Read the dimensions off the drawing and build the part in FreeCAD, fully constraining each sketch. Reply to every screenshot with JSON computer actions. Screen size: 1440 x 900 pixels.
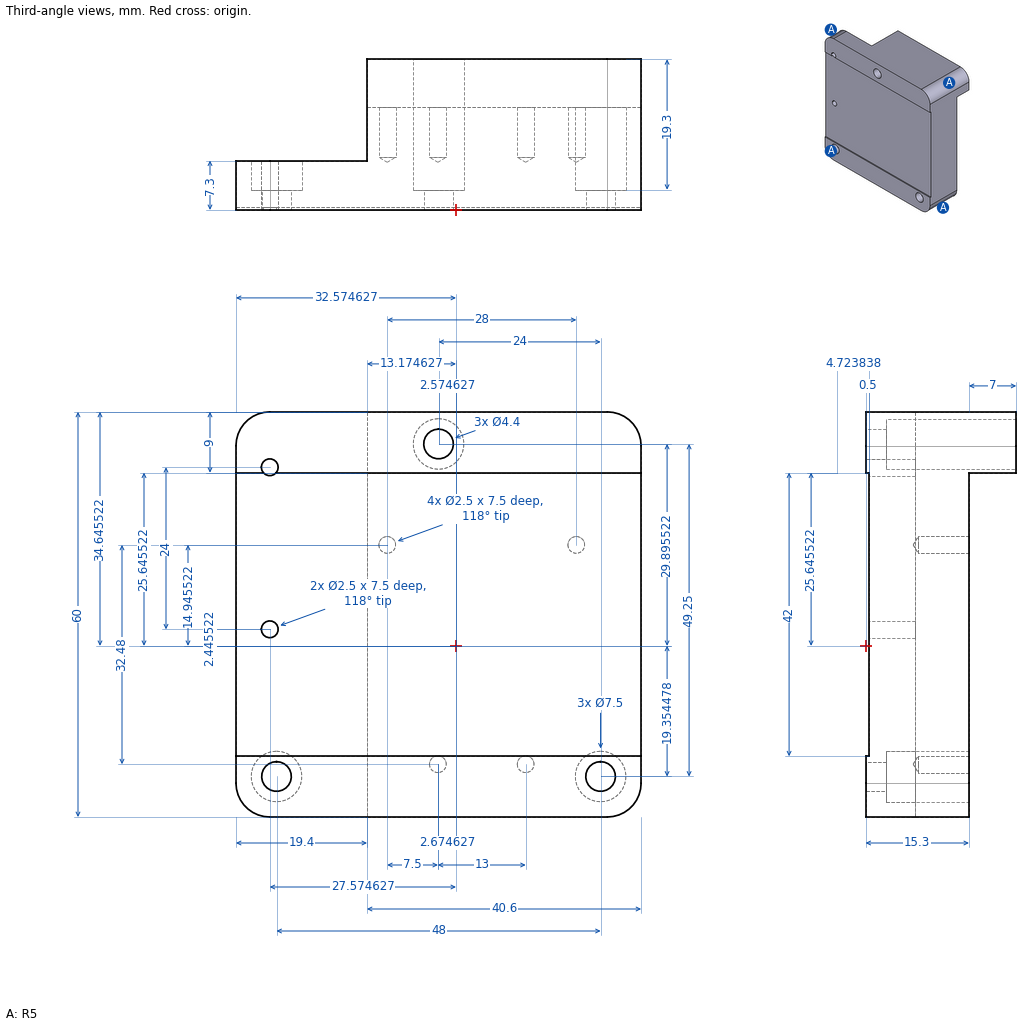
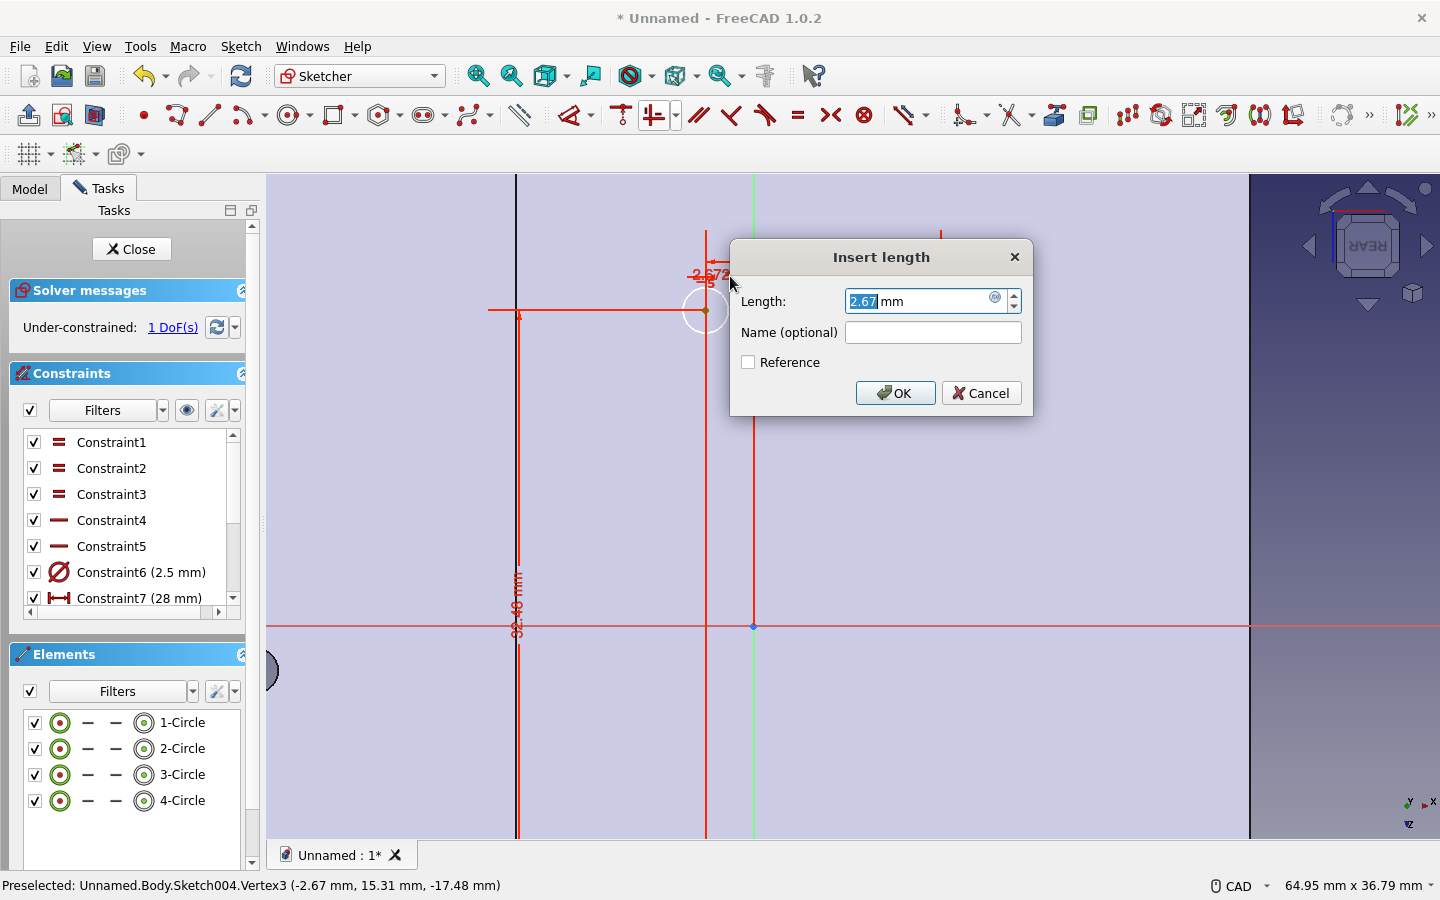
{"action": "type", "text": "2.674627"}
{"action": "key", "text": "Return"}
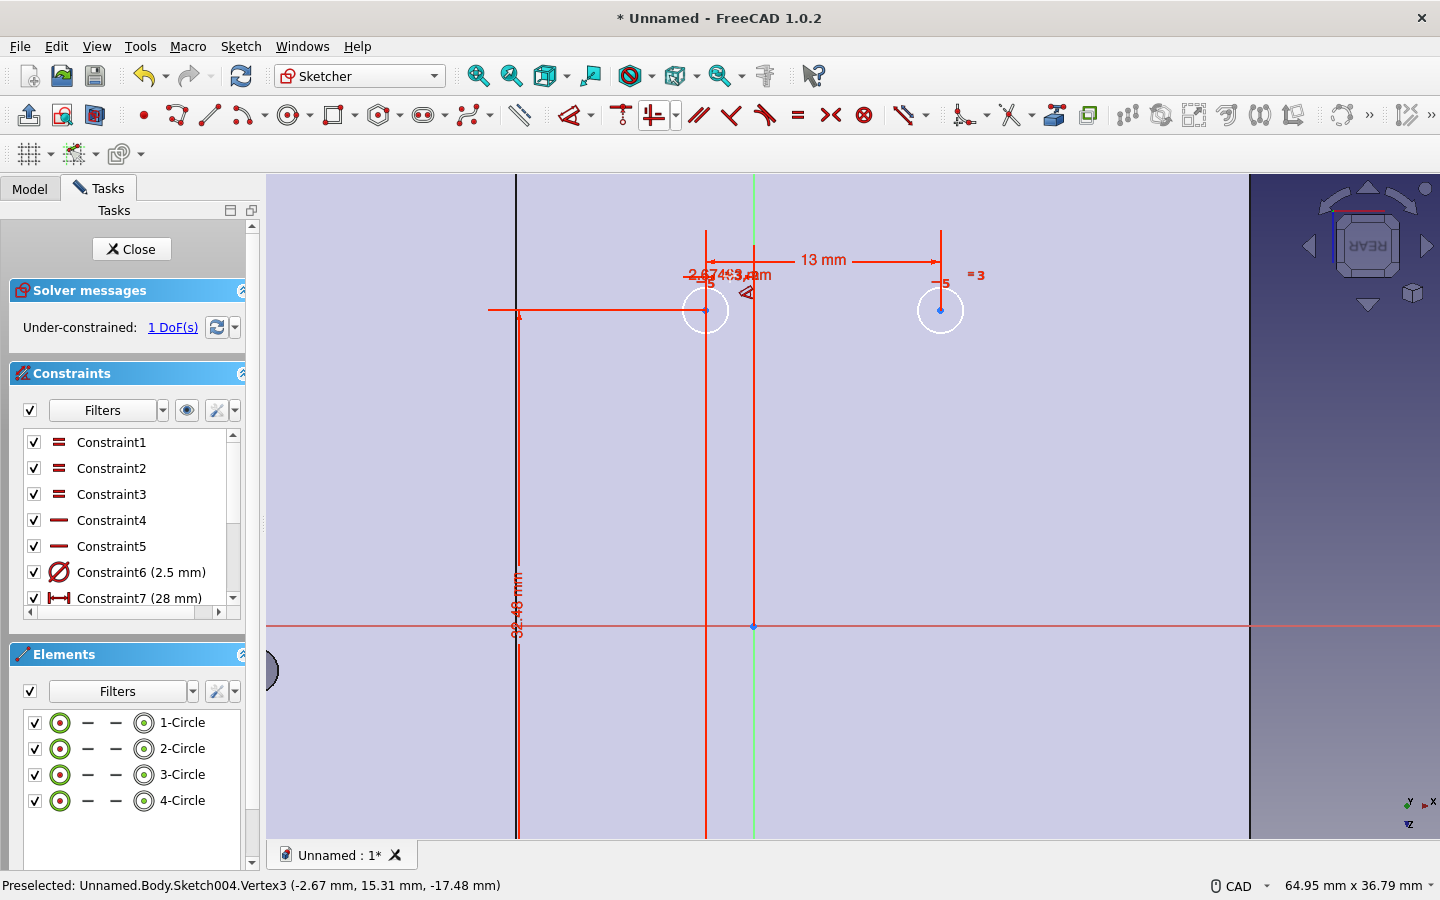
{"action": "scroll", "coordinate": [706, 310], "scroll_direction": "down", "scroll_amount": 2}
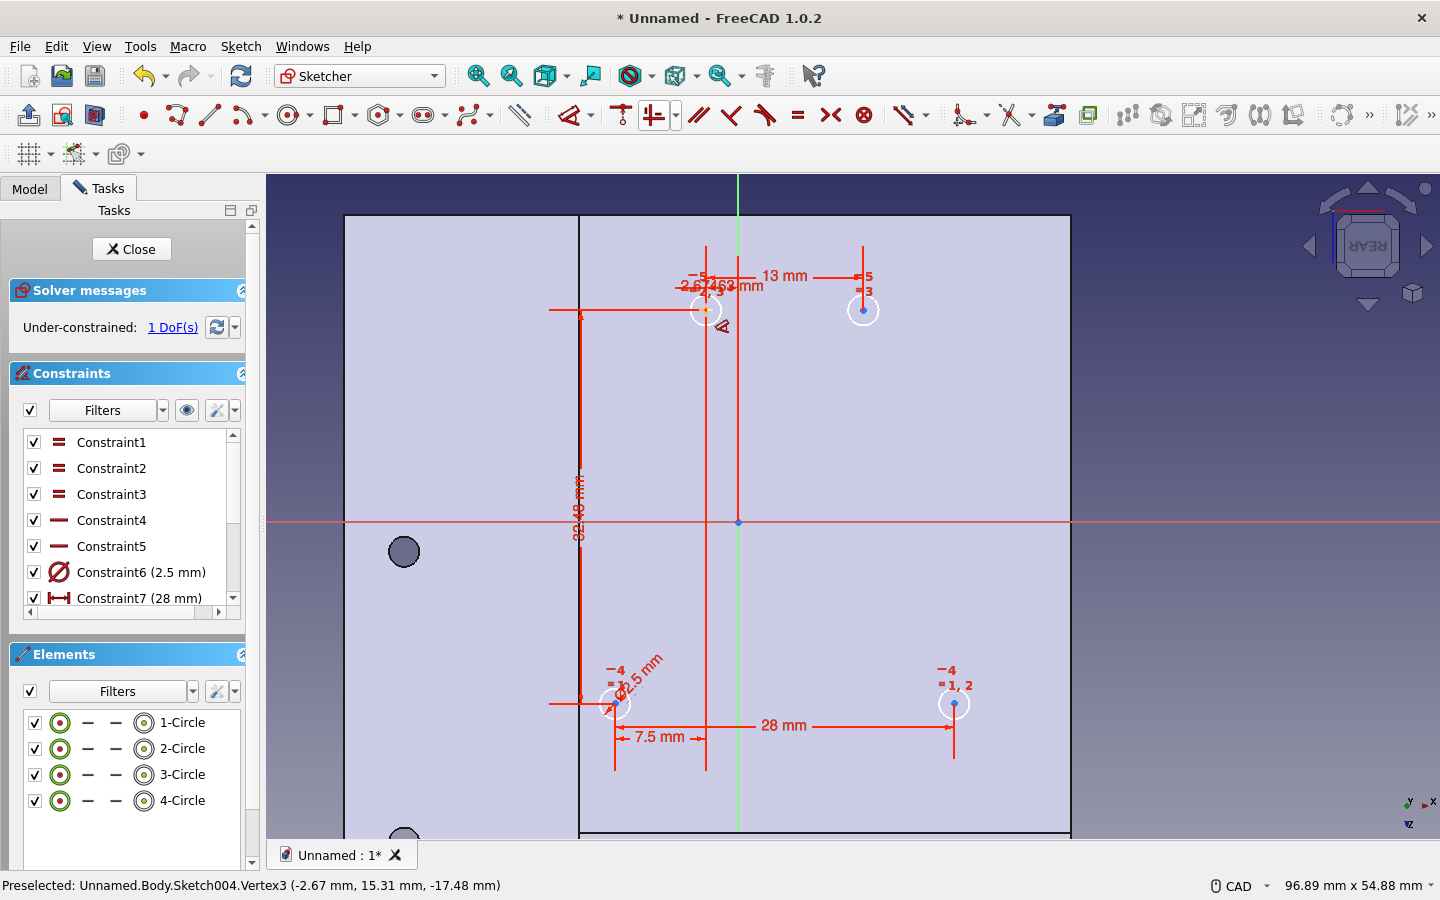
{"action": "left_click", "coordinate": [615, 704]}
{"action": "left_click", "coordinate": [581, 613]}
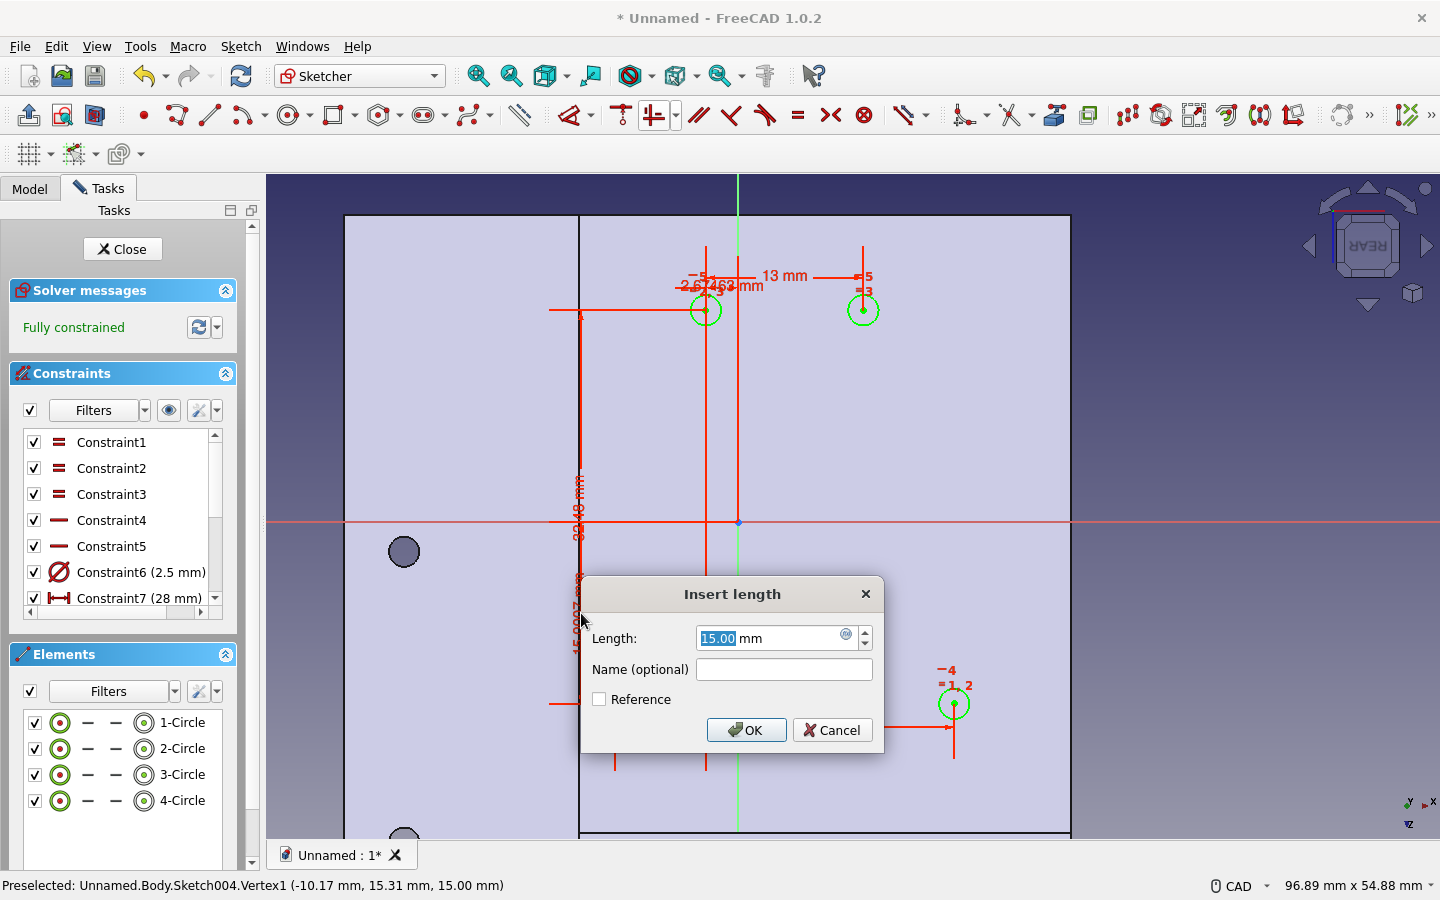
{"action": "type", "text": "14.945522"}
{"action": "key", "text": "Return"}
{"action": "key", "text": "Escape"}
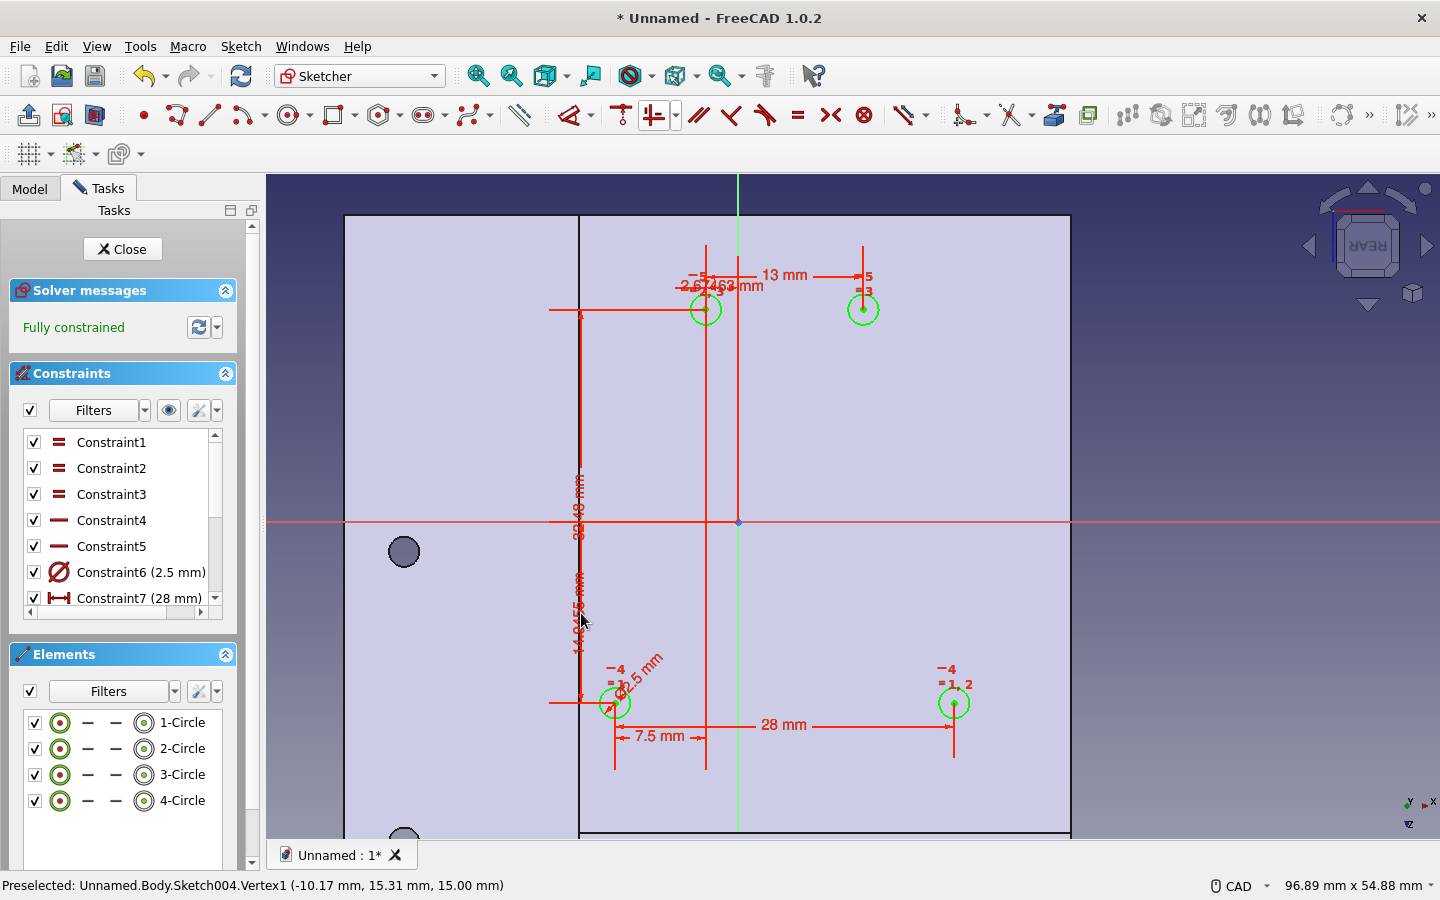
{"action": "left_click", "coordinate": [123, 249]}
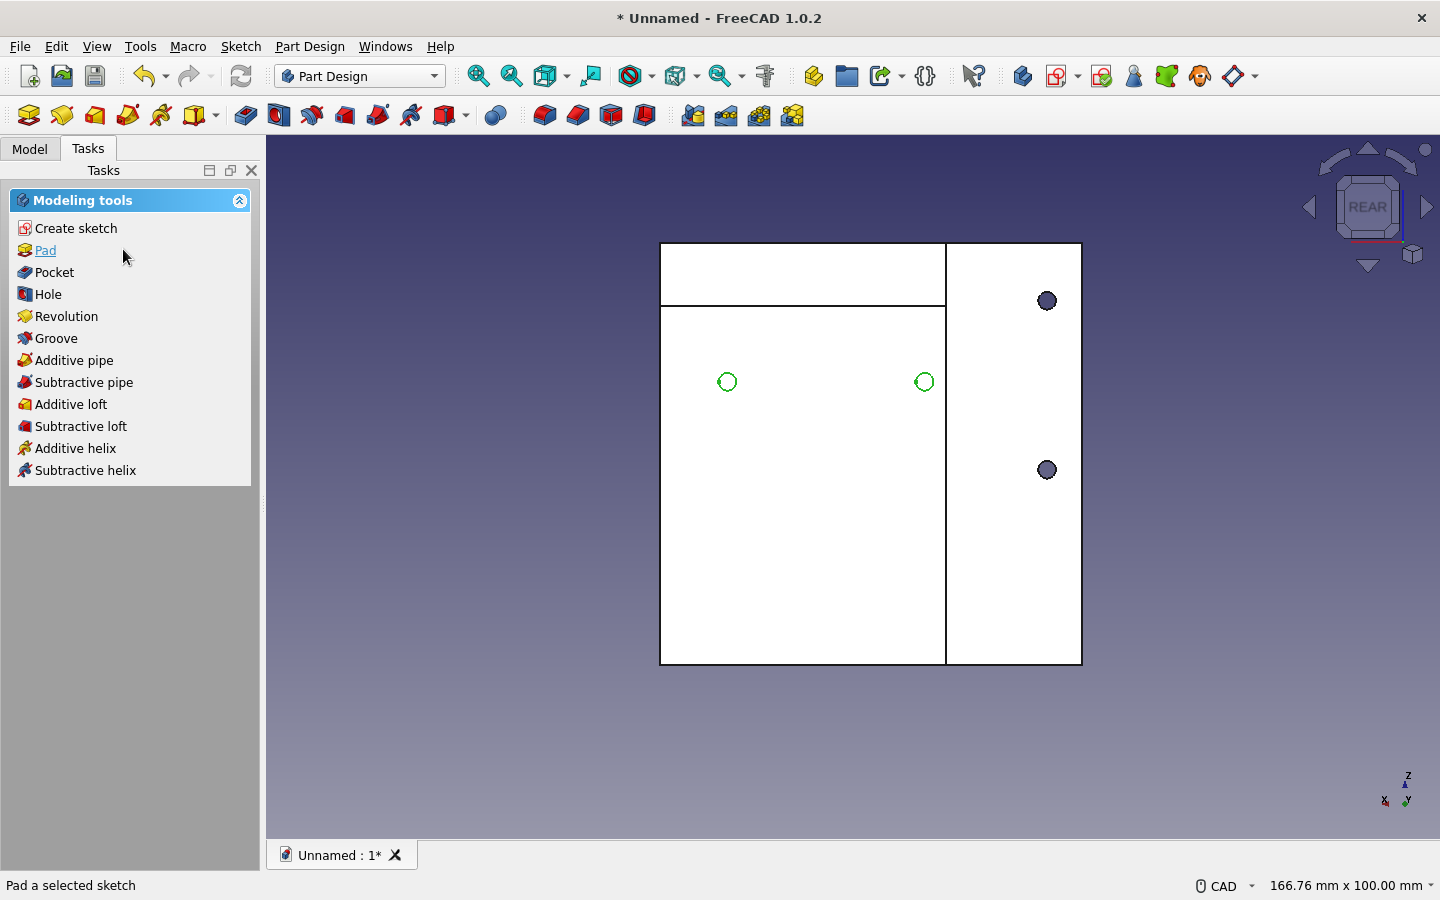
{"action": "left_click", "coordinate": [279, 116]}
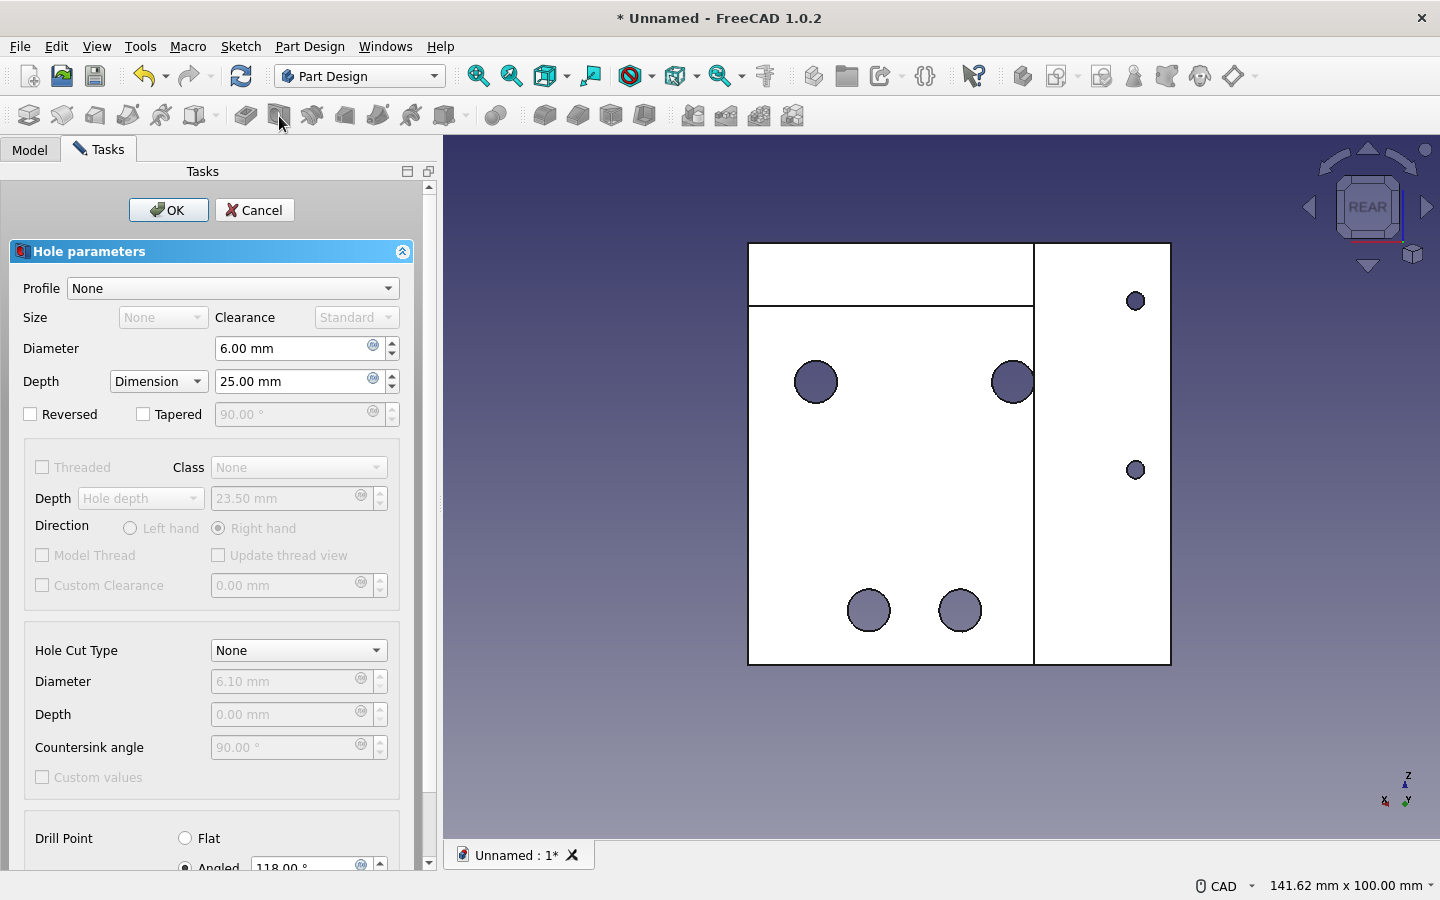
{"action": "triple_click", "coordinate": [300, 348]}